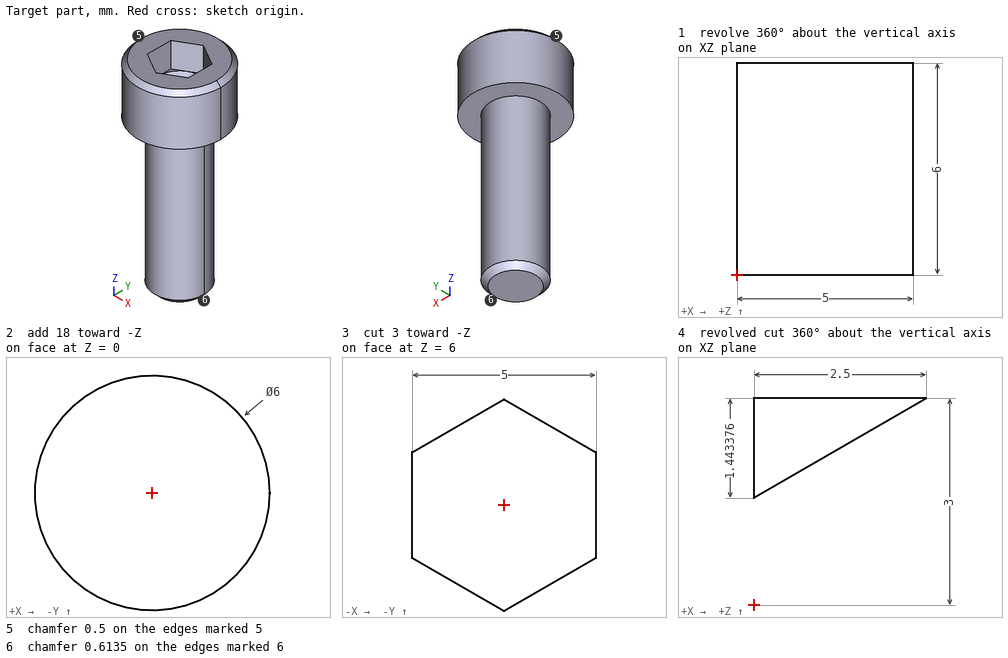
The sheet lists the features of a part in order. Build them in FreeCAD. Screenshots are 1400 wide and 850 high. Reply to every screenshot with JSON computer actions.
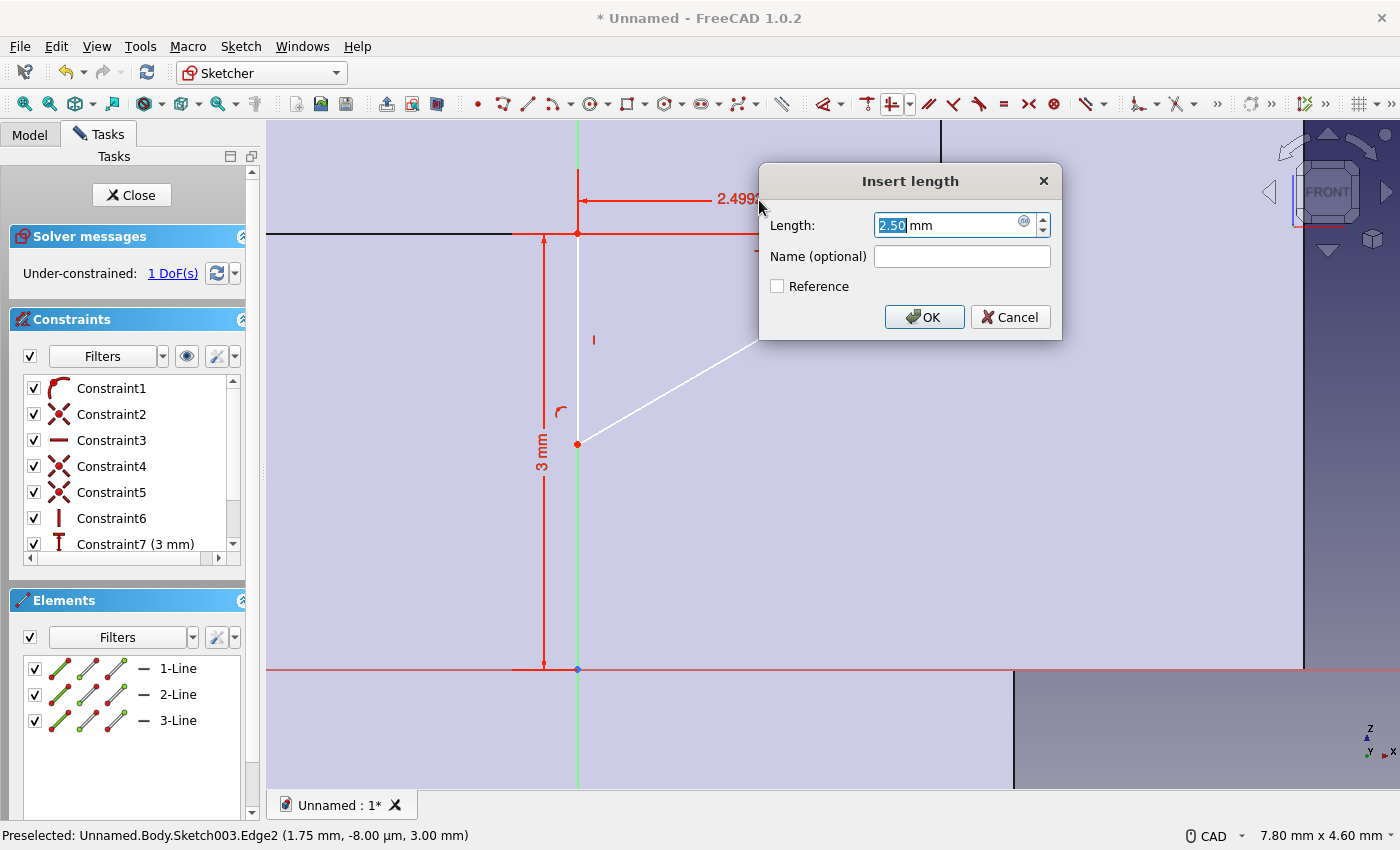
{"action": "type", "text": "2.5"}
{"action": "key", "text": "Return"}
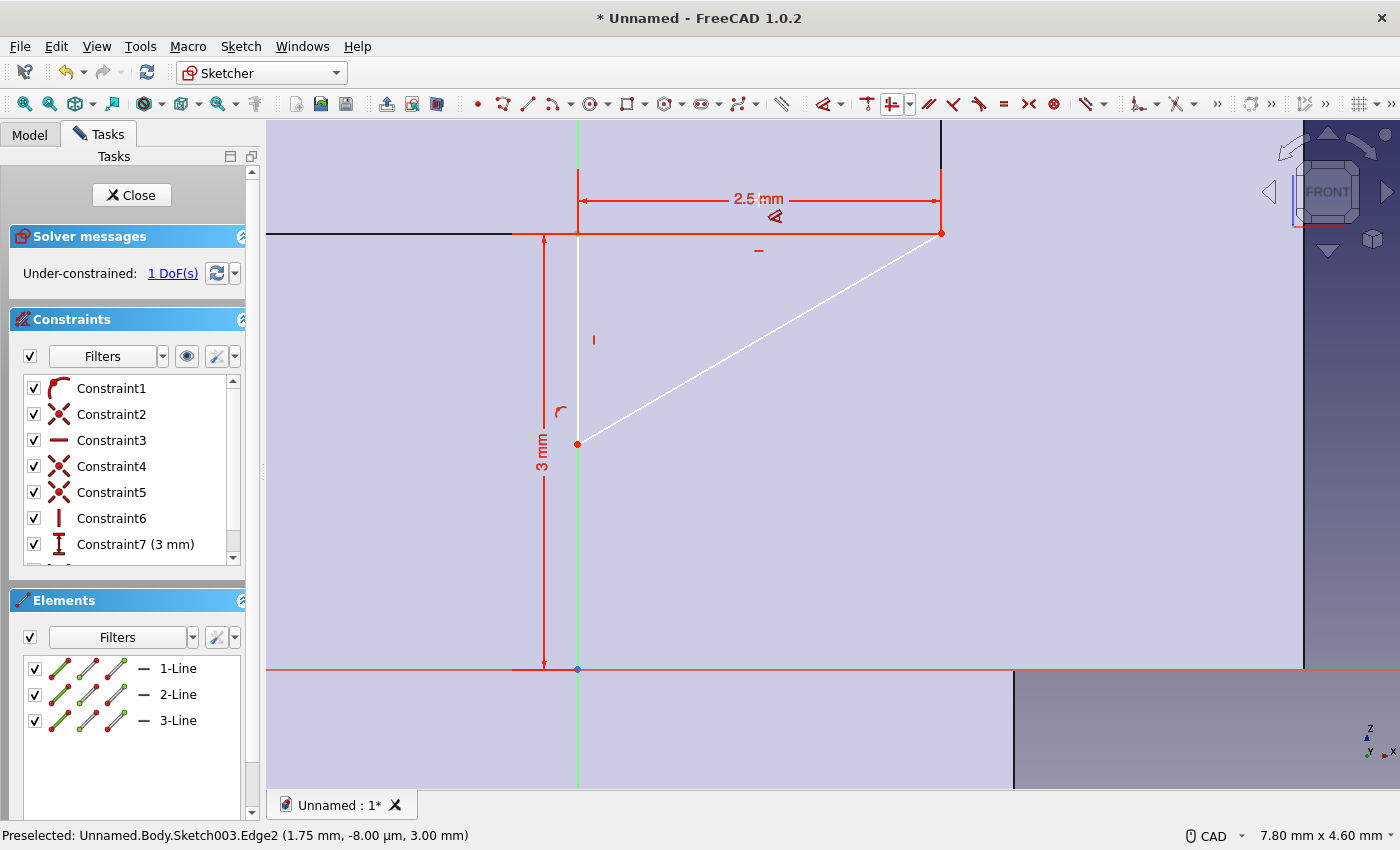
{"action": "left_click", "coordinate": [578, 297]}
{"action": "left_click", "coordinate": [544, 339]}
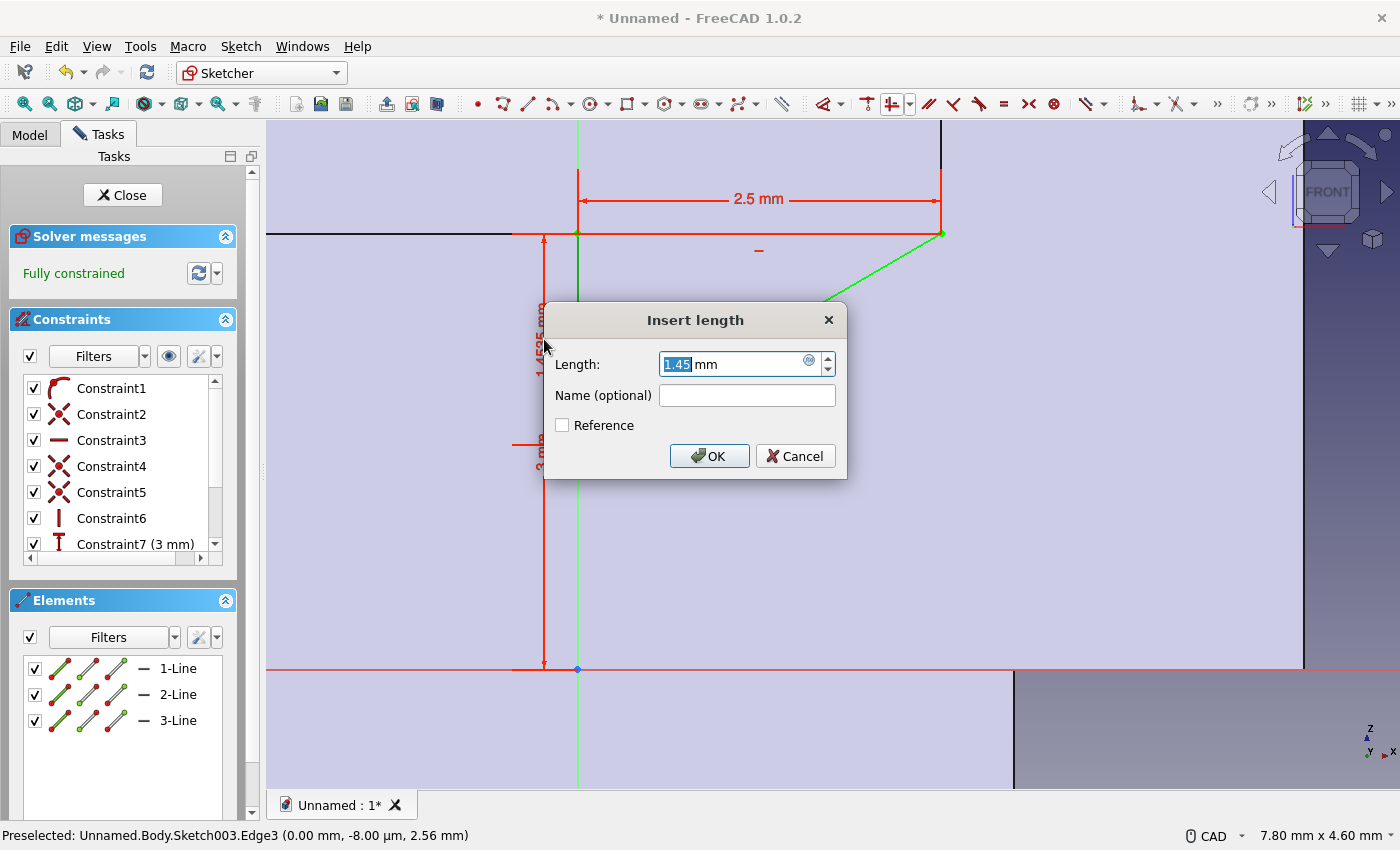
{"action": "type", "text": "1.443376"}
{"action": "key", "text": "Return"}
{"action": "key", "text": "Escape"}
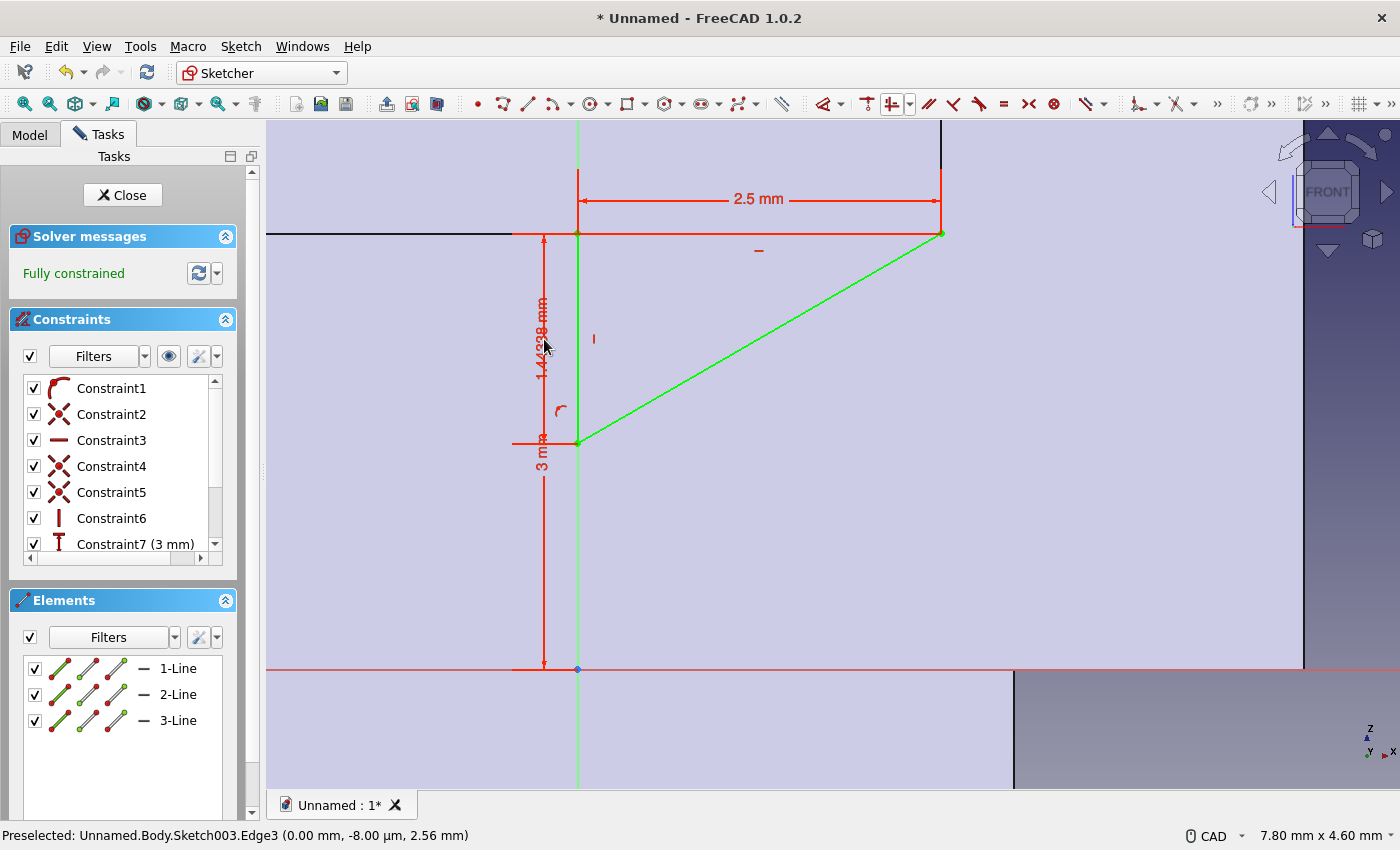
{"action": "left_click", "coordinate": [123, 195]}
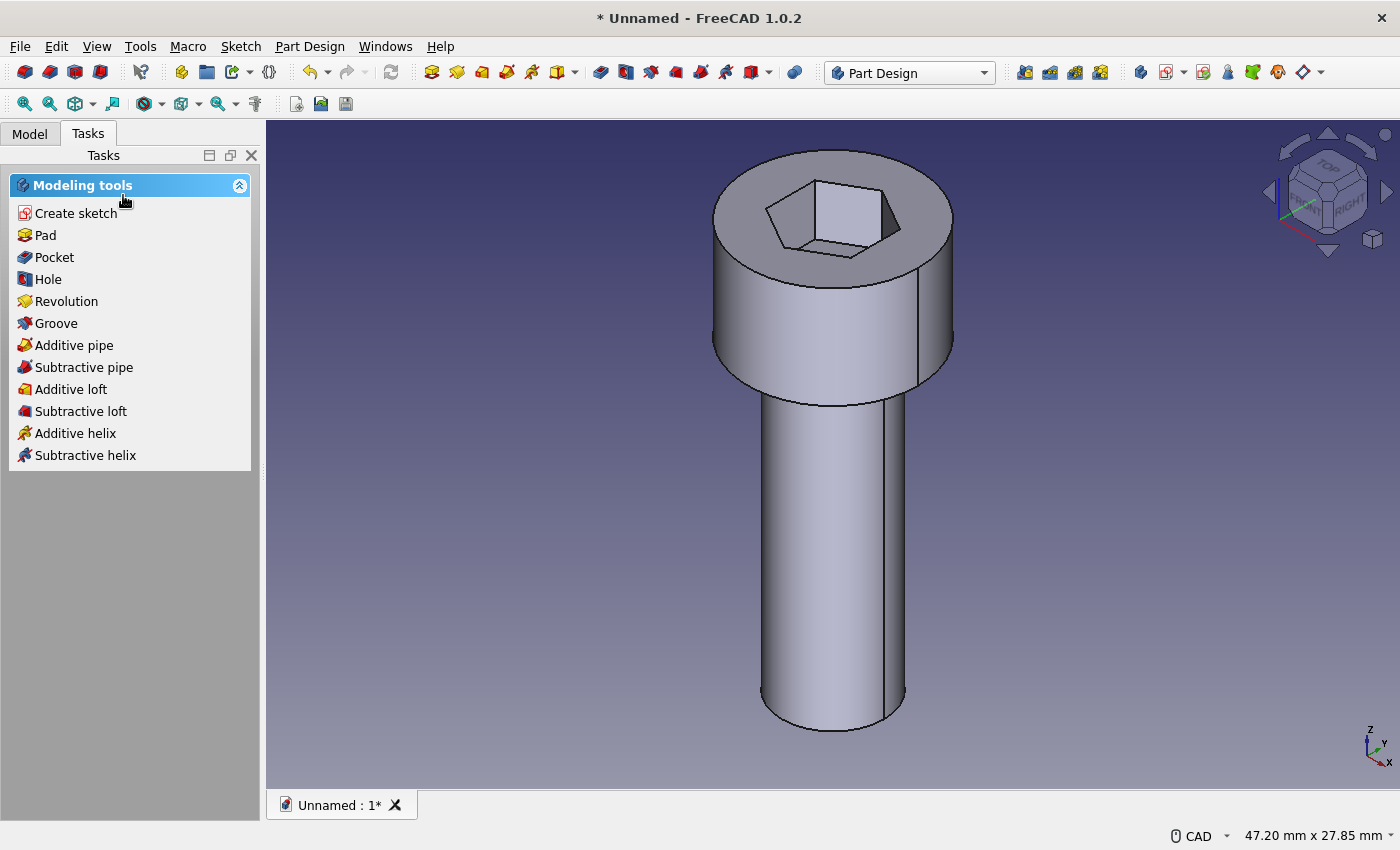
{"action": "left_click", "coordinate": [651, 72]}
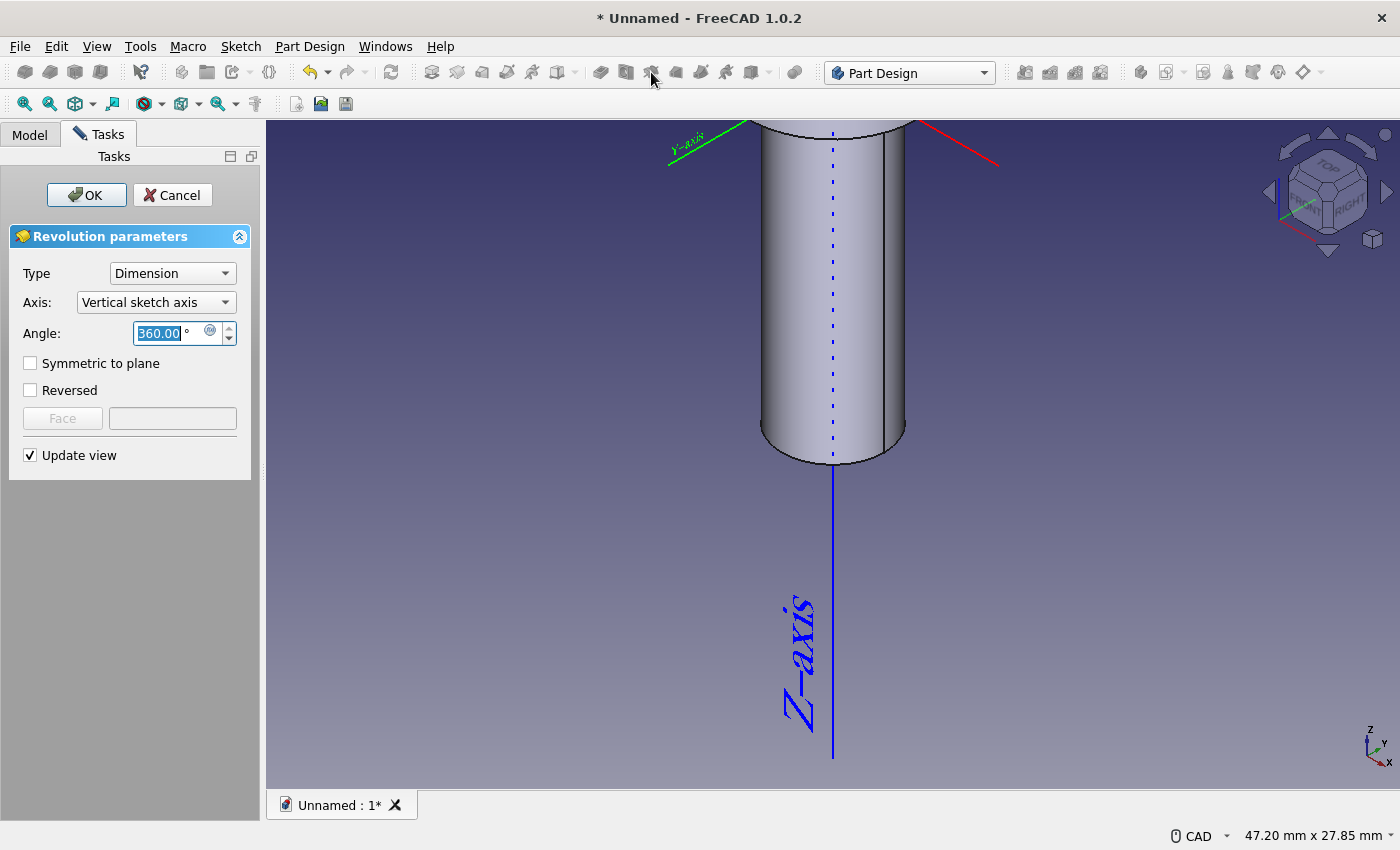
{"action": "left_click", "coordinate": [87, 195]}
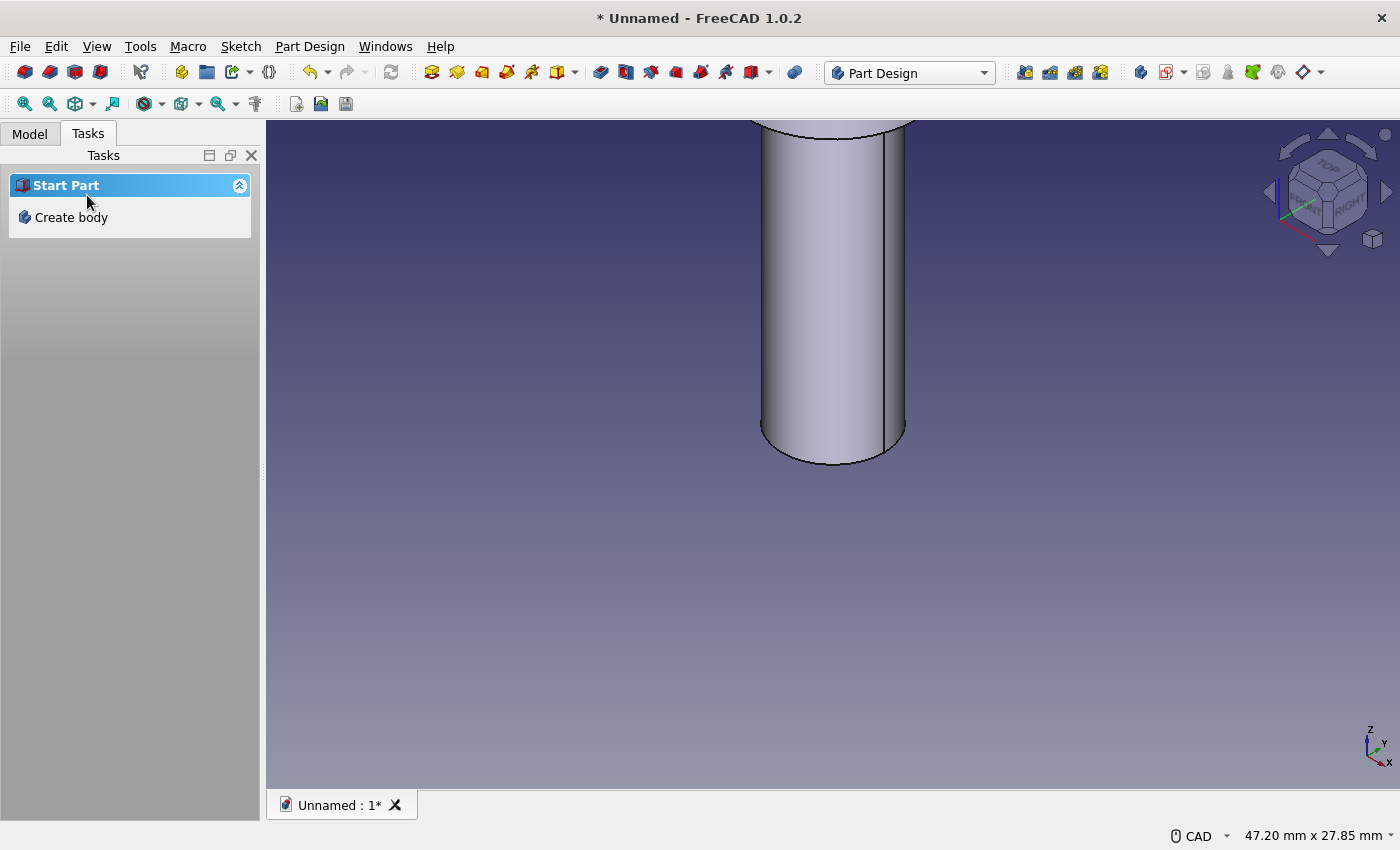
{"action": "left_click", "coordinate": [25, 104]}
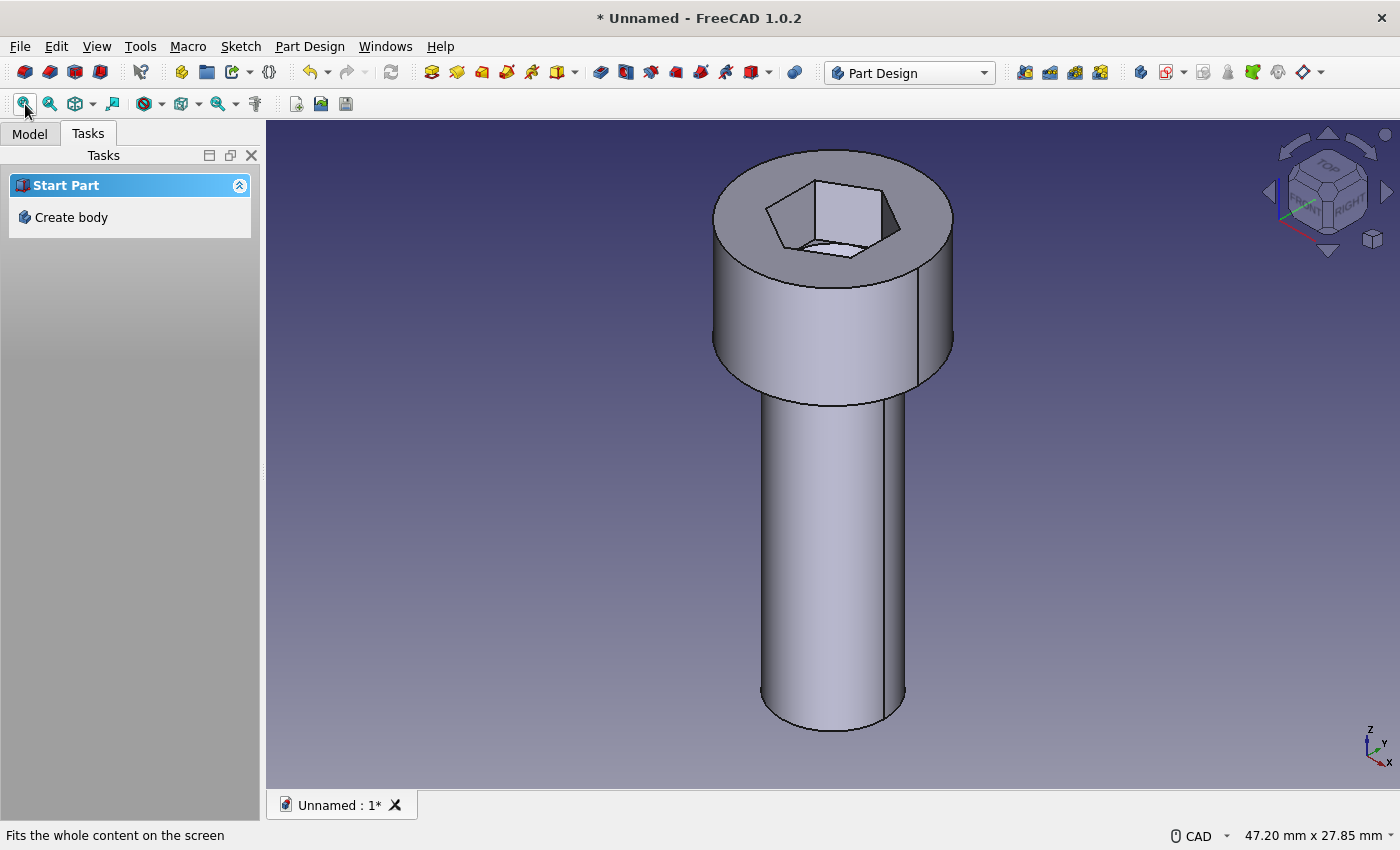
{"action": "left_click", "coordinate": [726, 250]}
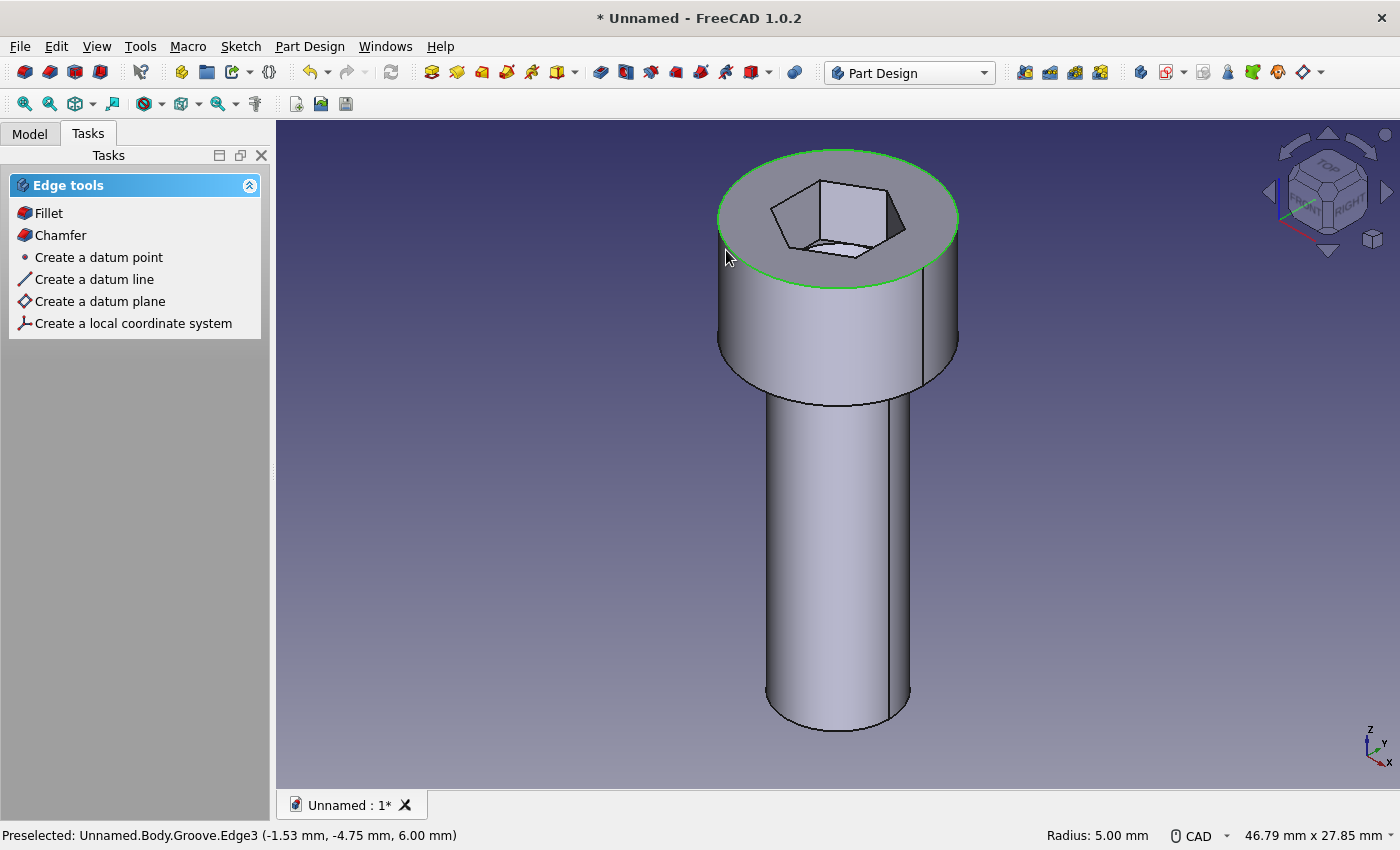
{"action": "left_click", "coordinate": [50, 72]}